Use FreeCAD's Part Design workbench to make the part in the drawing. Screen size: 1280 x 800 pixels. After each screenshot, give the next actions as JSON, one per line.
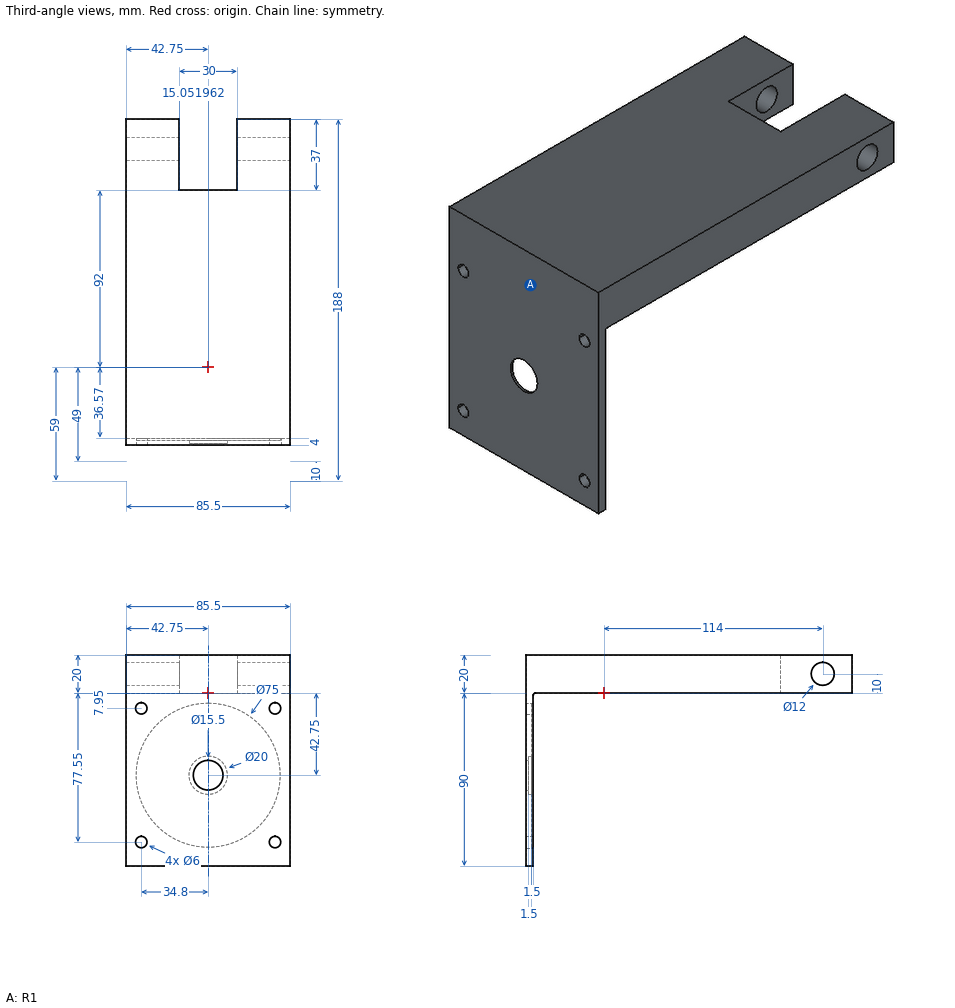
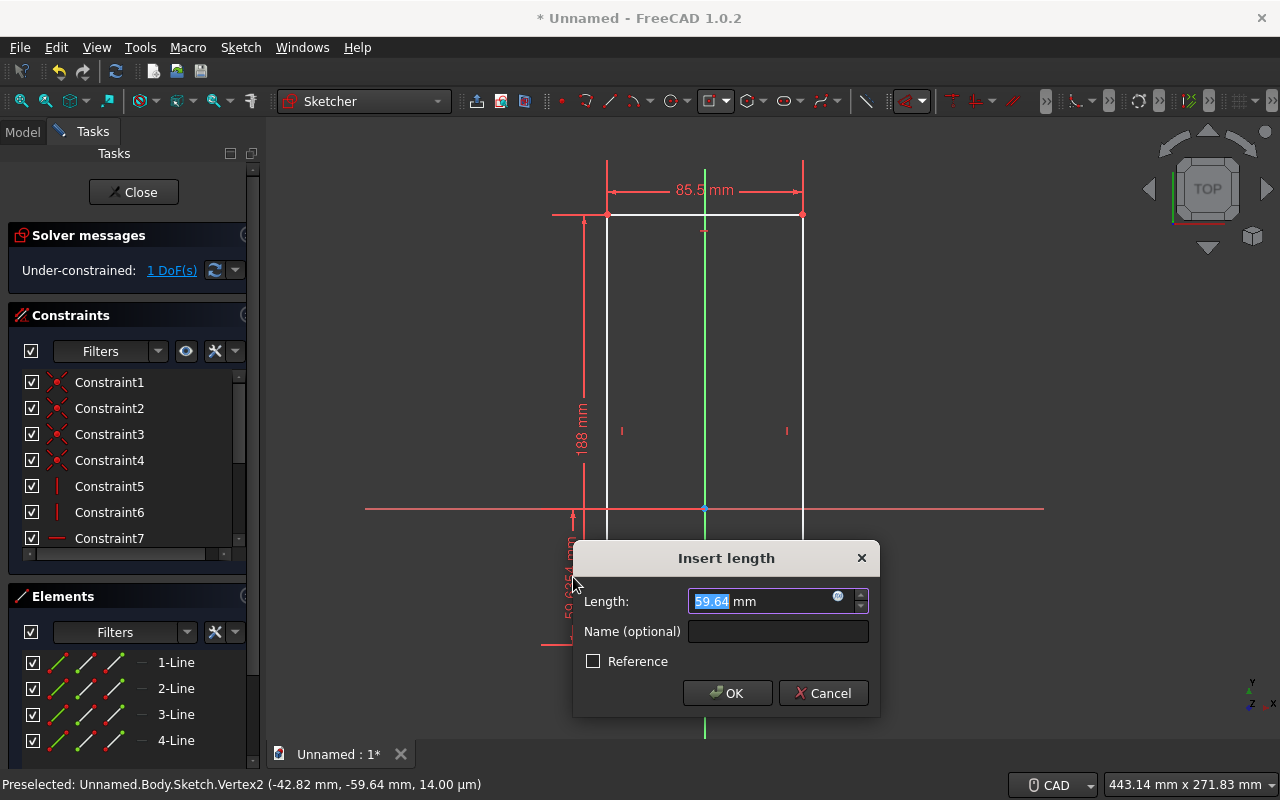
{"action": "type", "text": "59"}
{"action": "key", "text": "Return"}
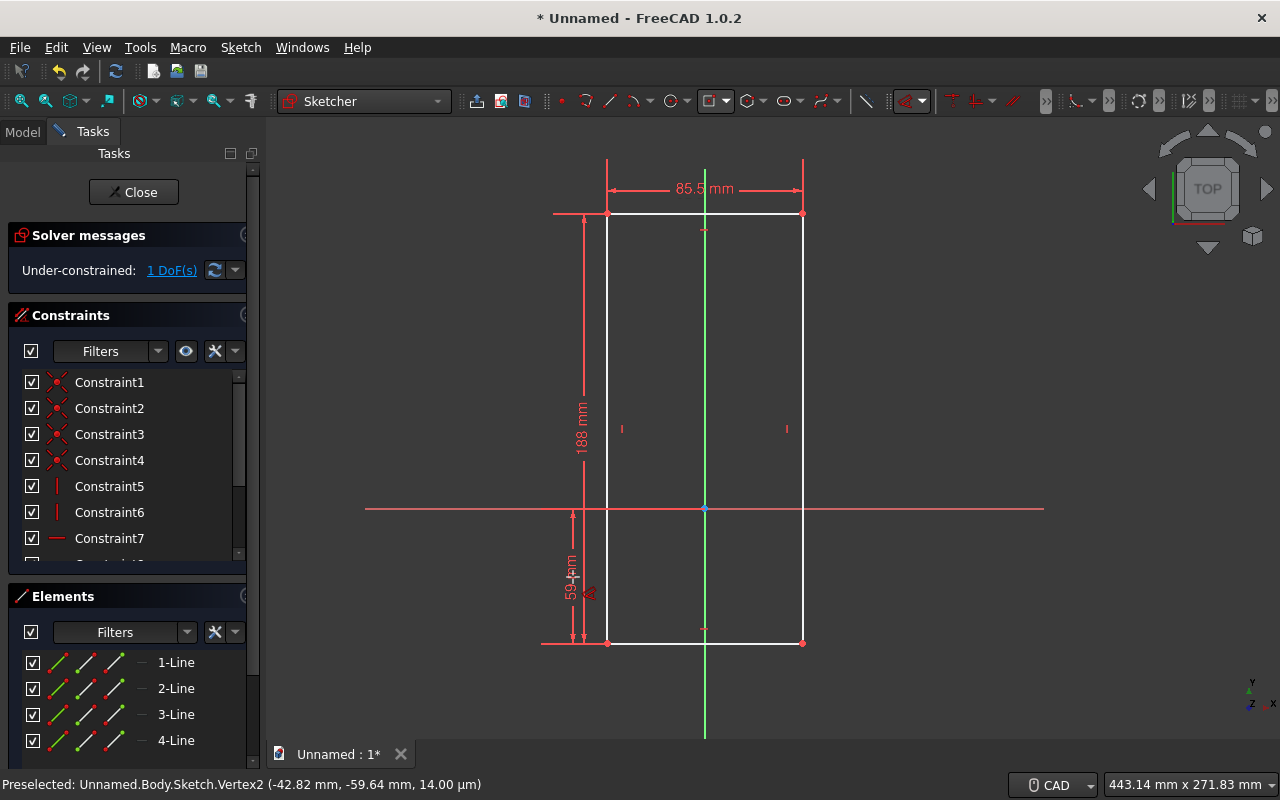
{"action": "left_click", "coordinate": [607, 214]}
{"action": "left_click", "coordinate": [656, 180]}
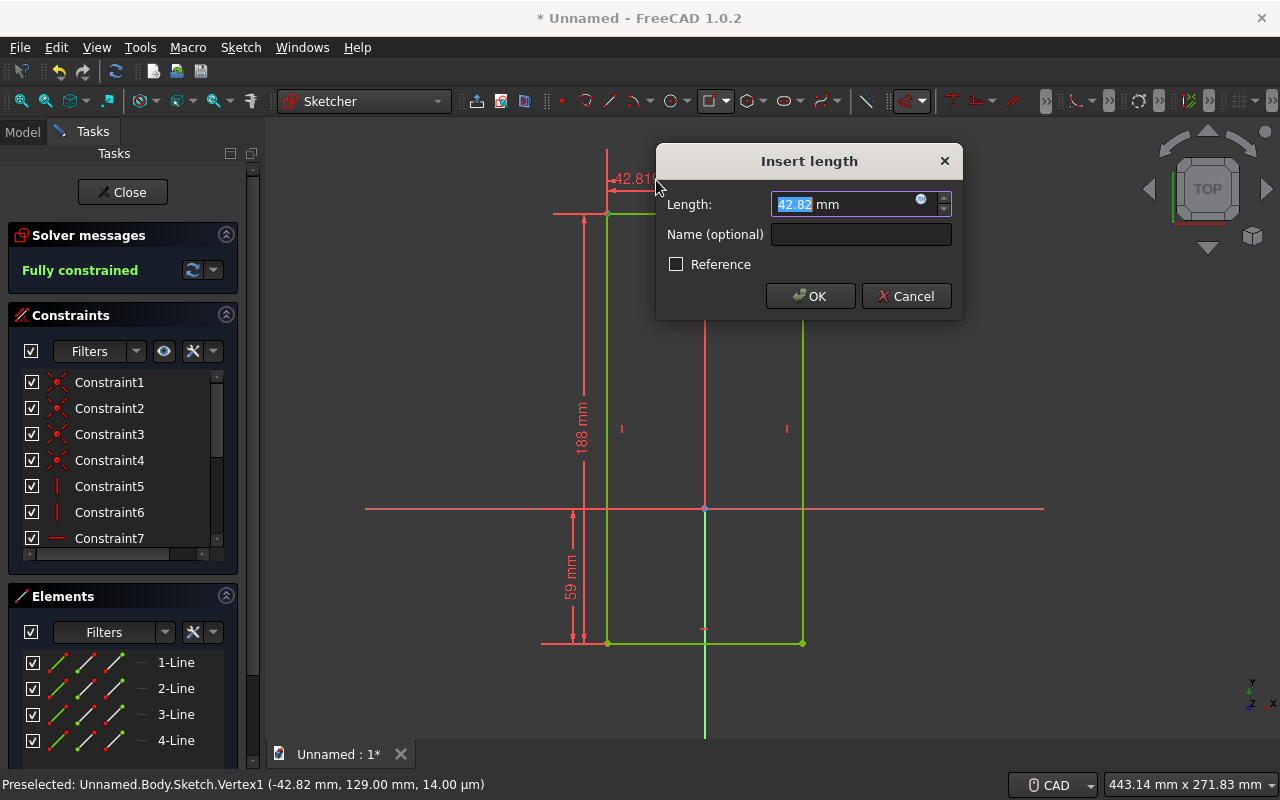
{"action": "type", "text": "42.75"}
{"action": "key", "text": "Return"}
{"action": "key", "text": "Escape"}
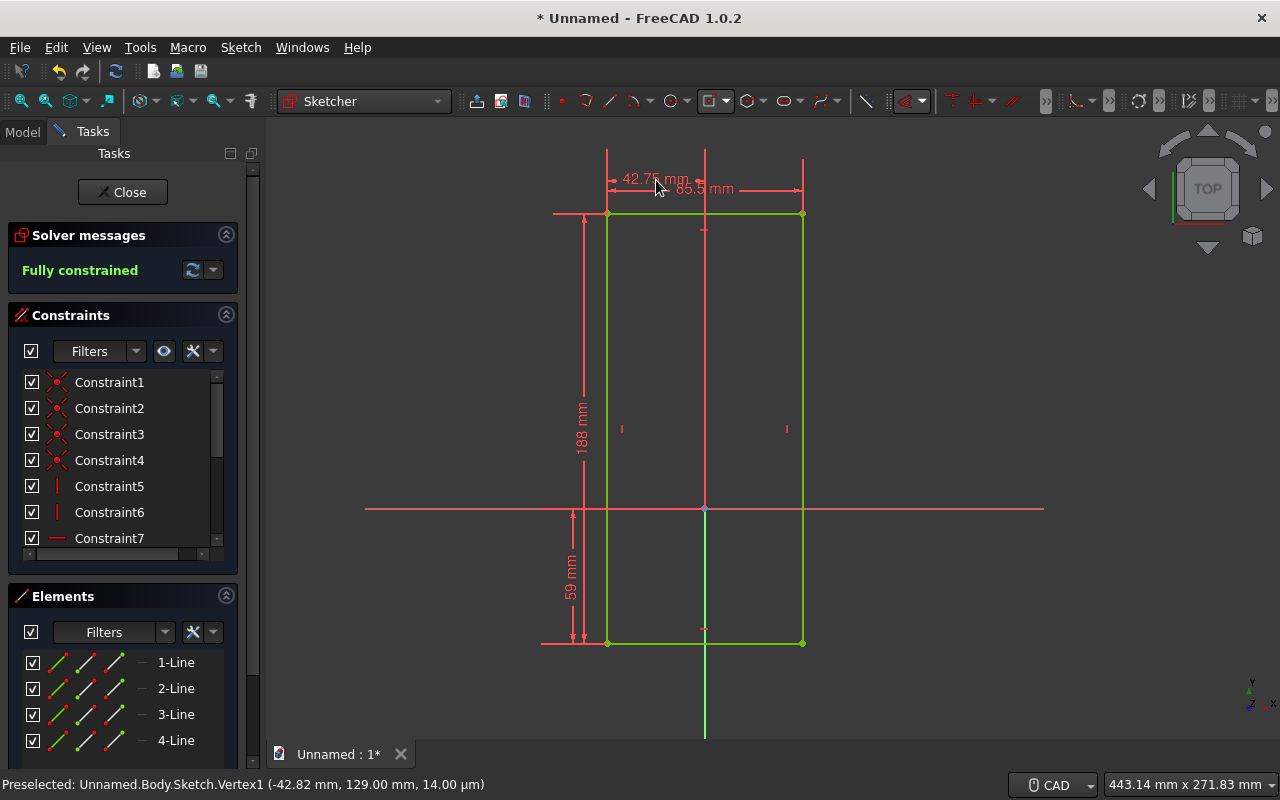
{"action": "left_click", "coordinate": [123, 192]}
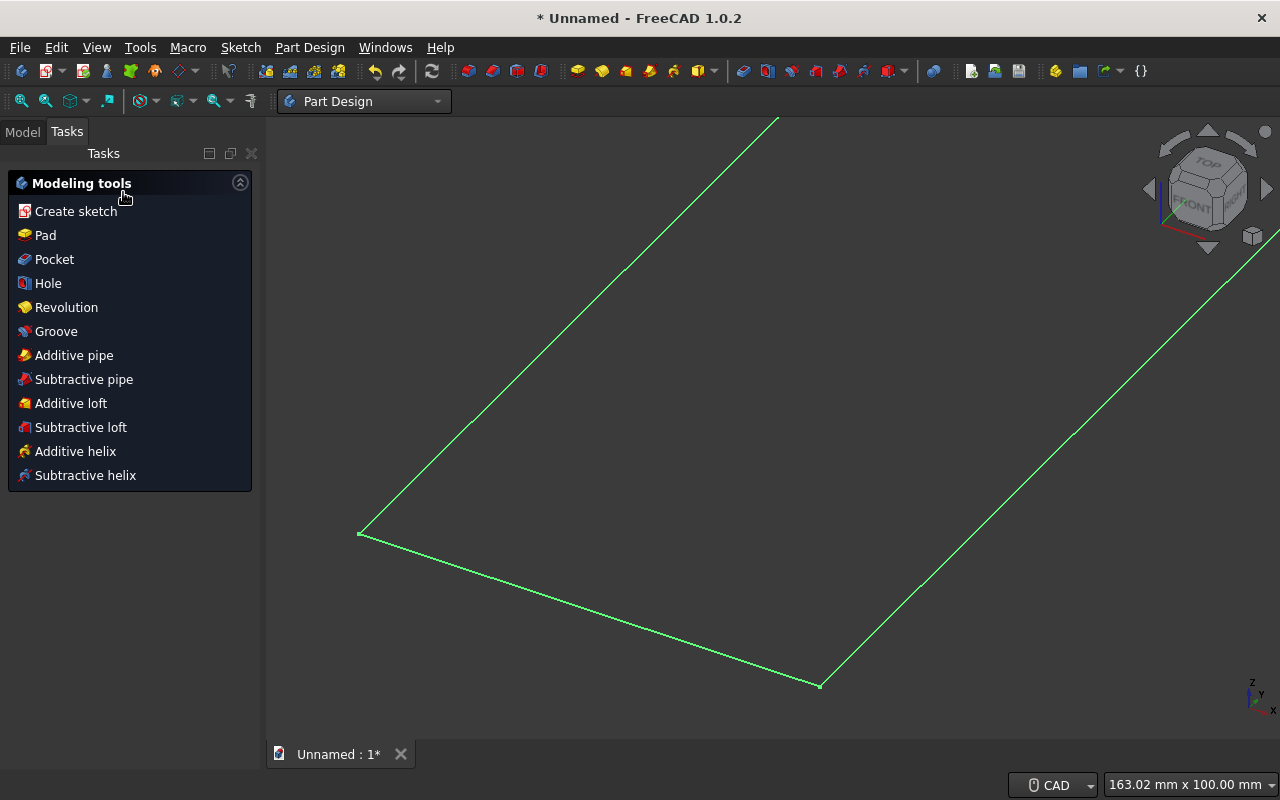
{"action": "left_click", "coordinate": [578, 72]}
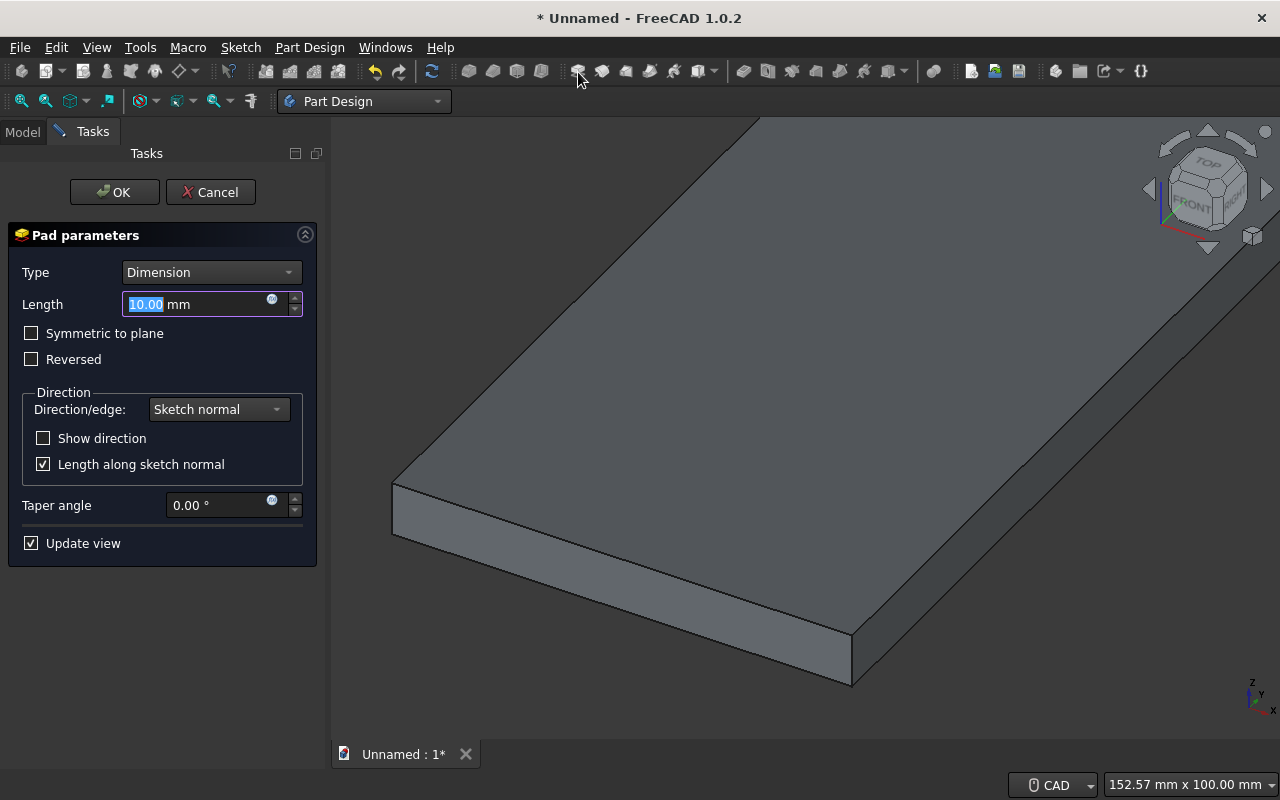
{"action": "type", "text": "20"}
{"action": "key", "text": "Tab"}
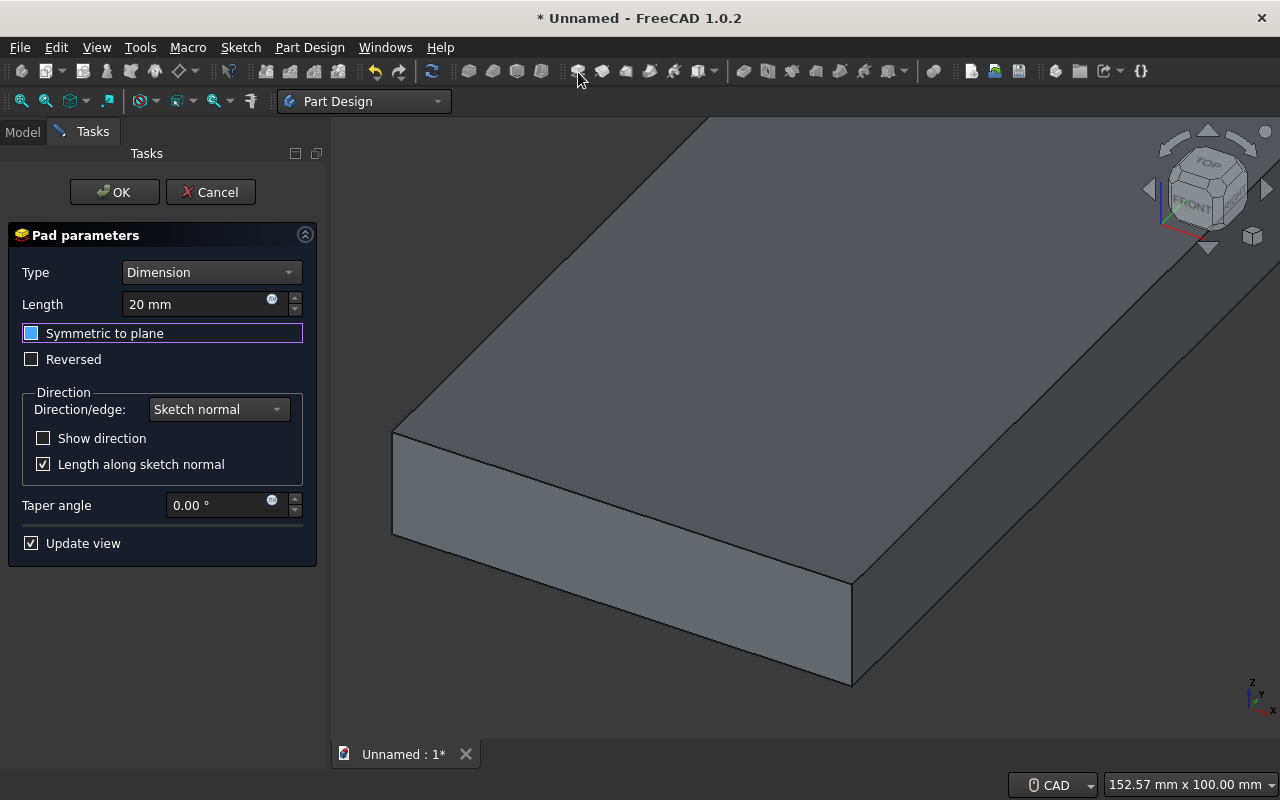
{"action": "left_click", "coordinate": [115, 192]}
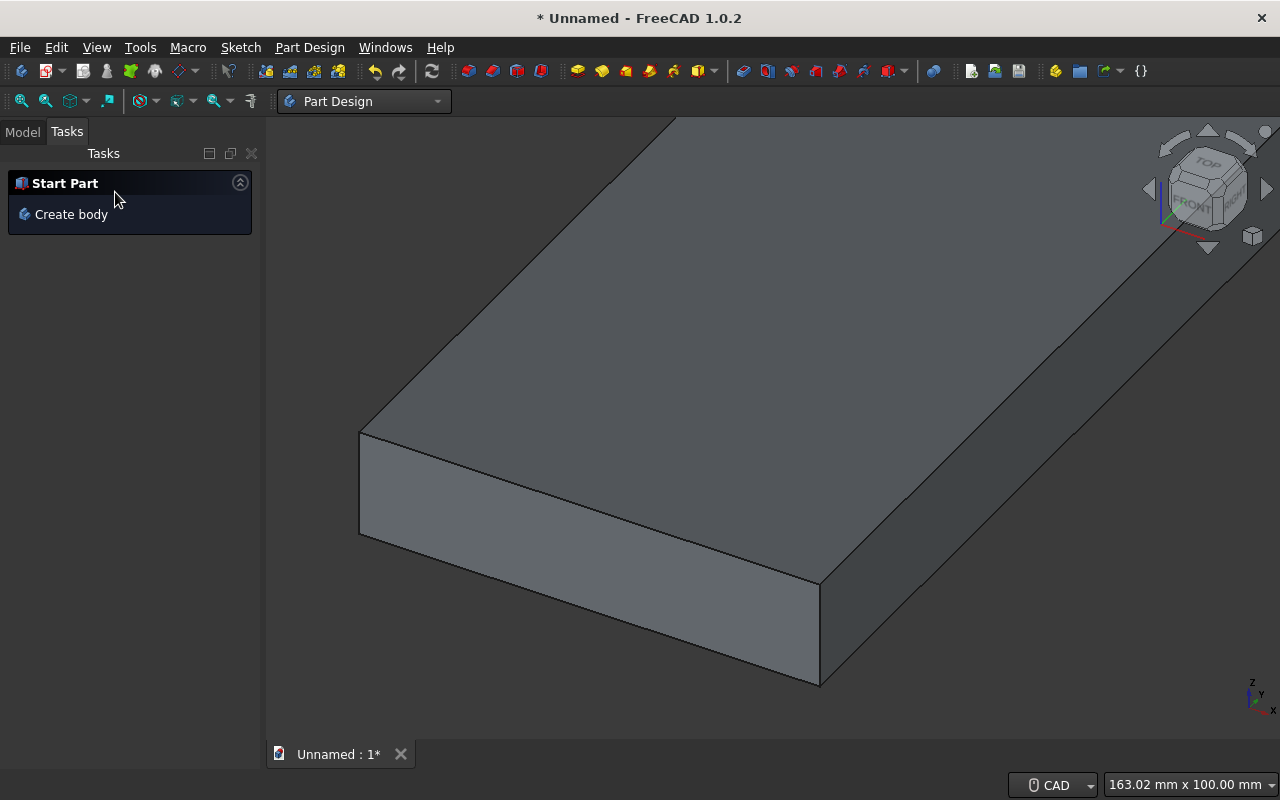
{"action": "left_click", "coordinate": [22, 102]}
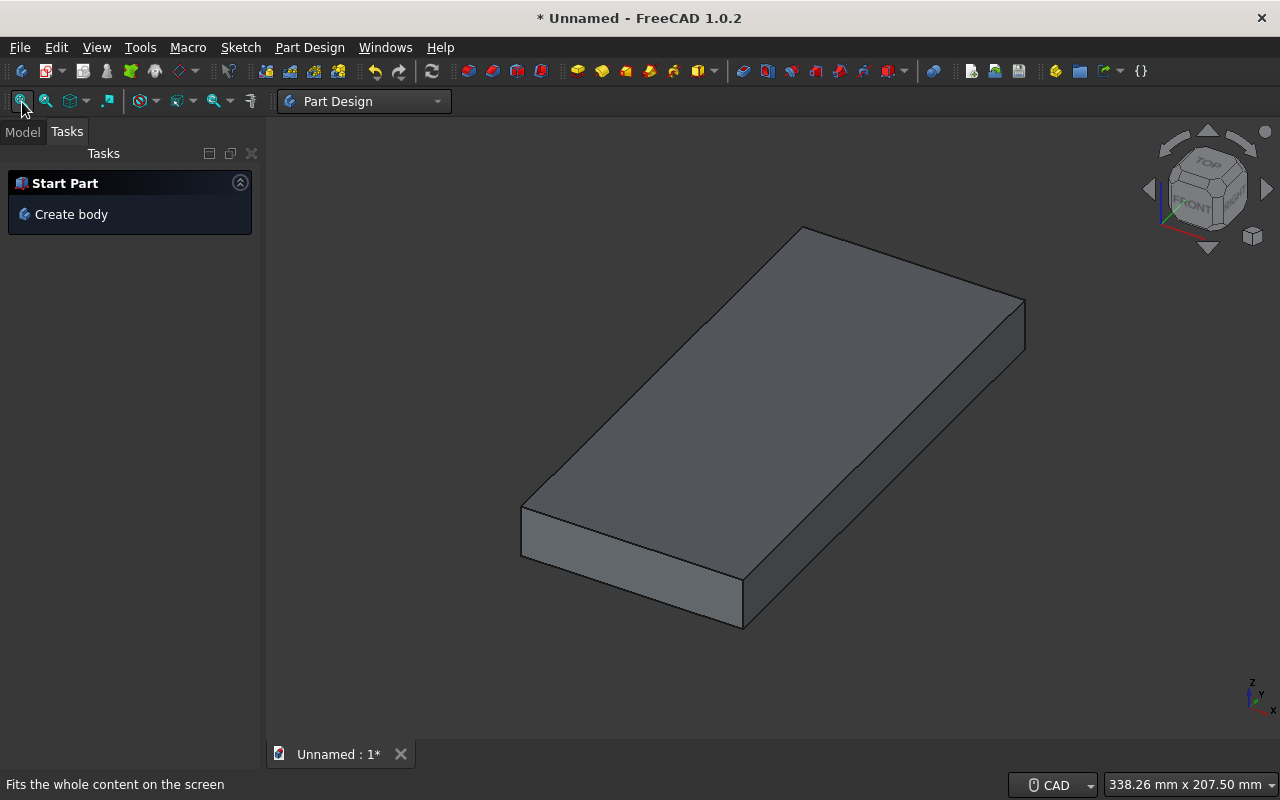
{"action": "left_click", "coordinate": [813, 362]}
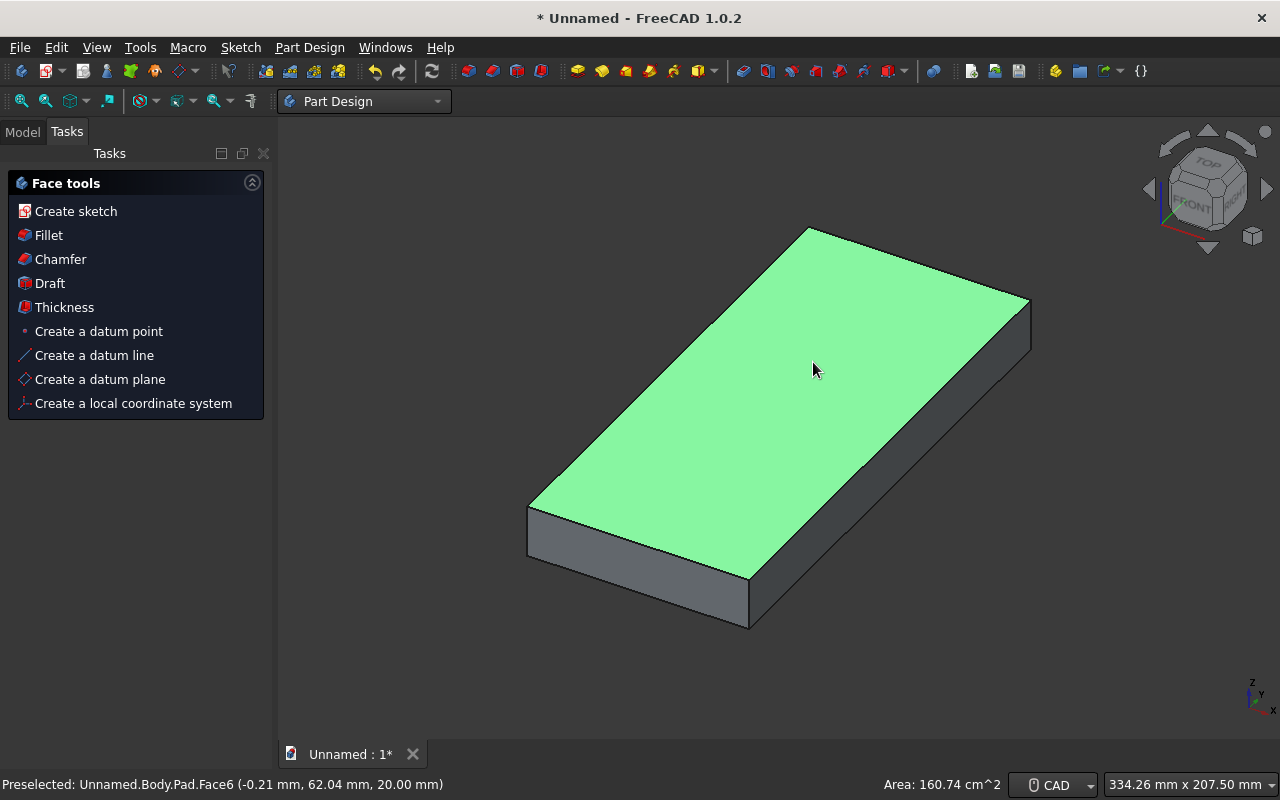
{"action": "left_click", "coordinate": [46, 72]}